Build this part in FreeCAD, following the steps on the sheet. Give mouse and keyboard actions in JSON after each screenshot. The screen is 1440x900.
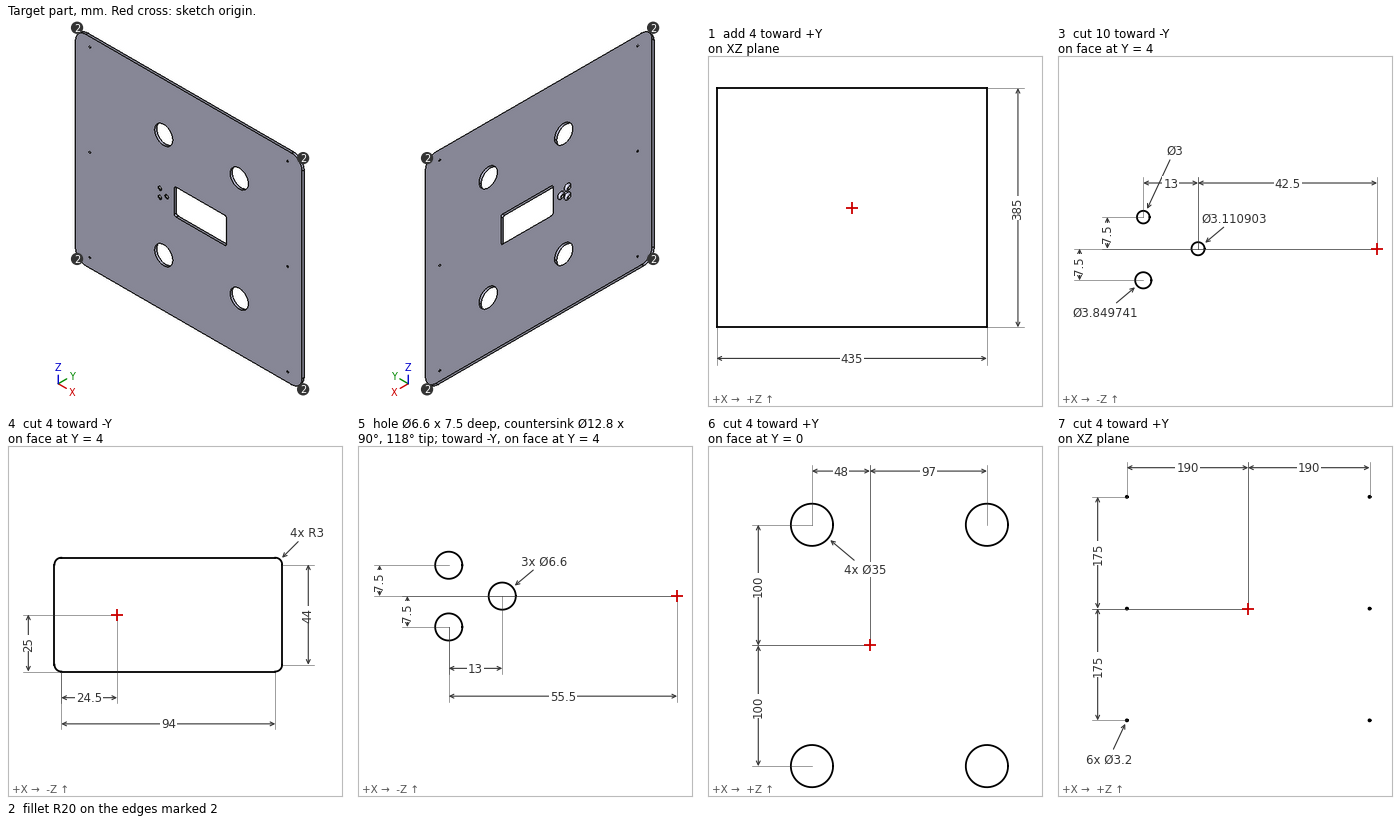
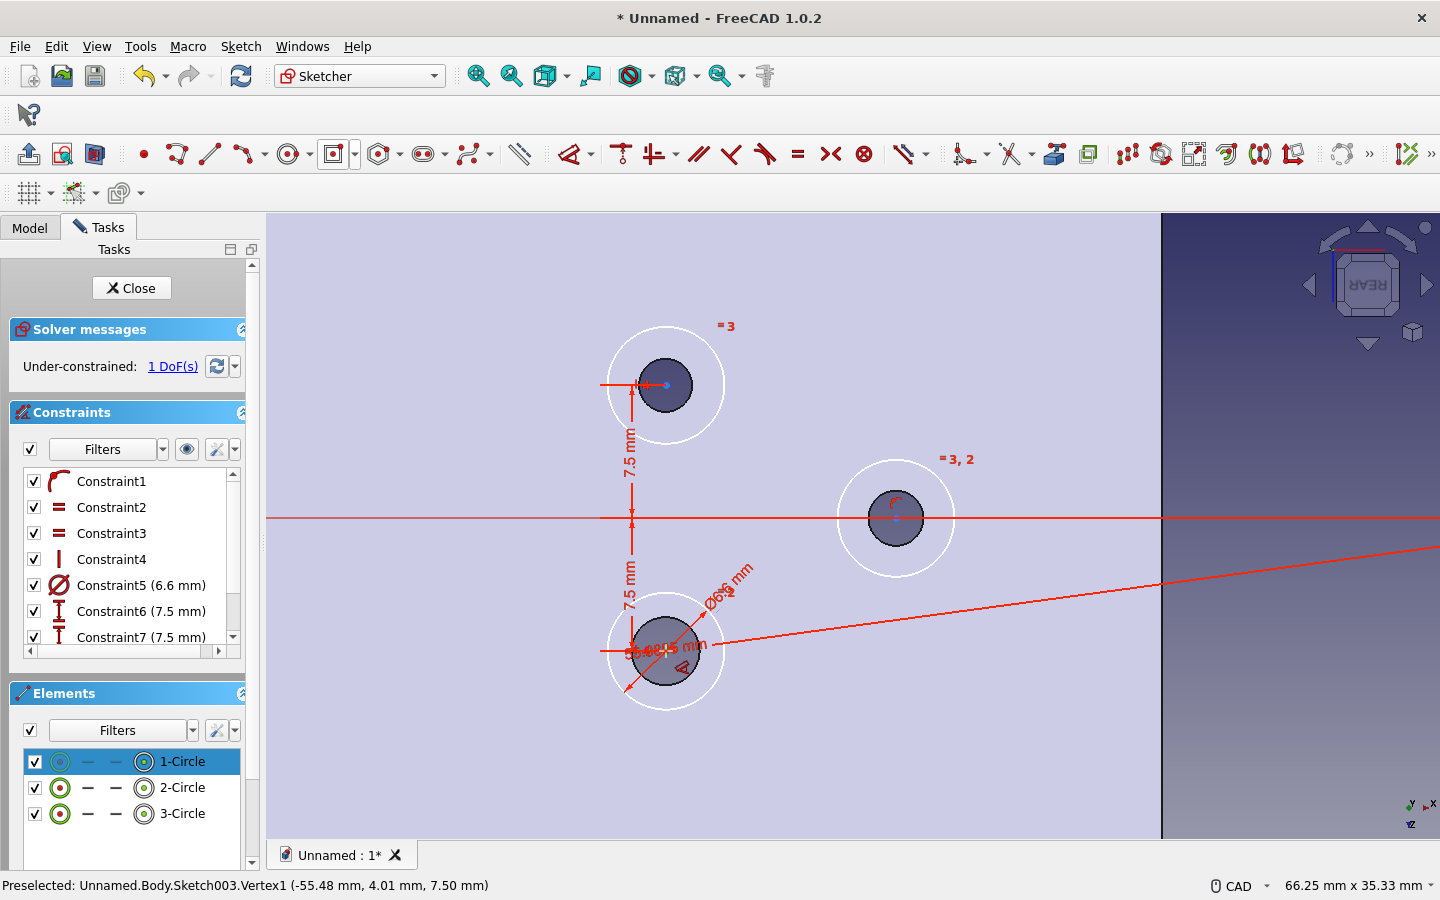
{"action": "left_click", "coordinate": [896, 518]}
{"action": "left_click", "coordinate": [781, 685]}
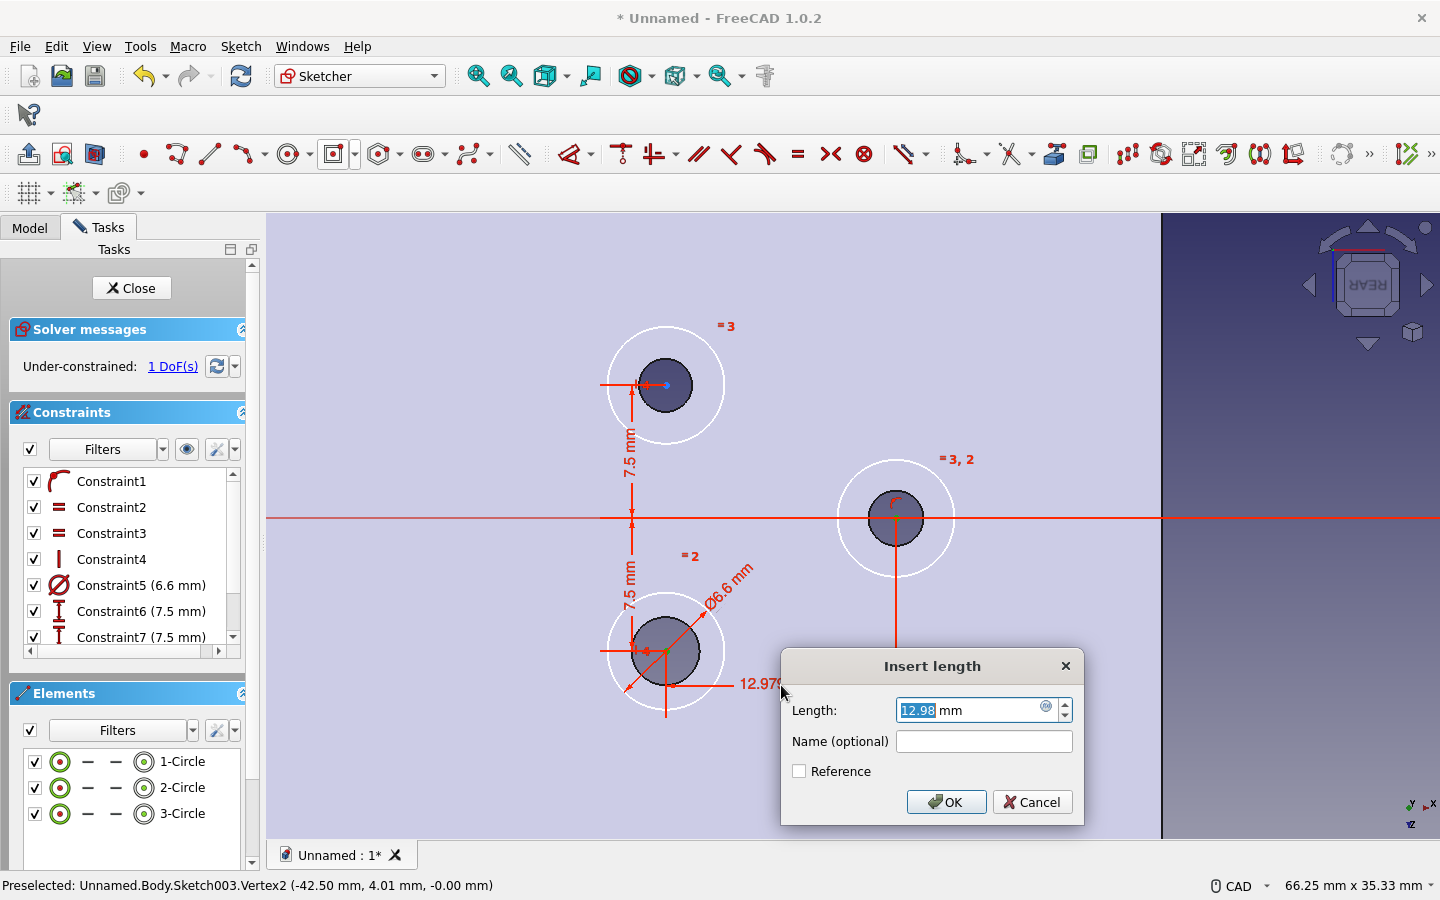
{"action": "type", "text": "13"}
{"action": "key", "text": "Return"}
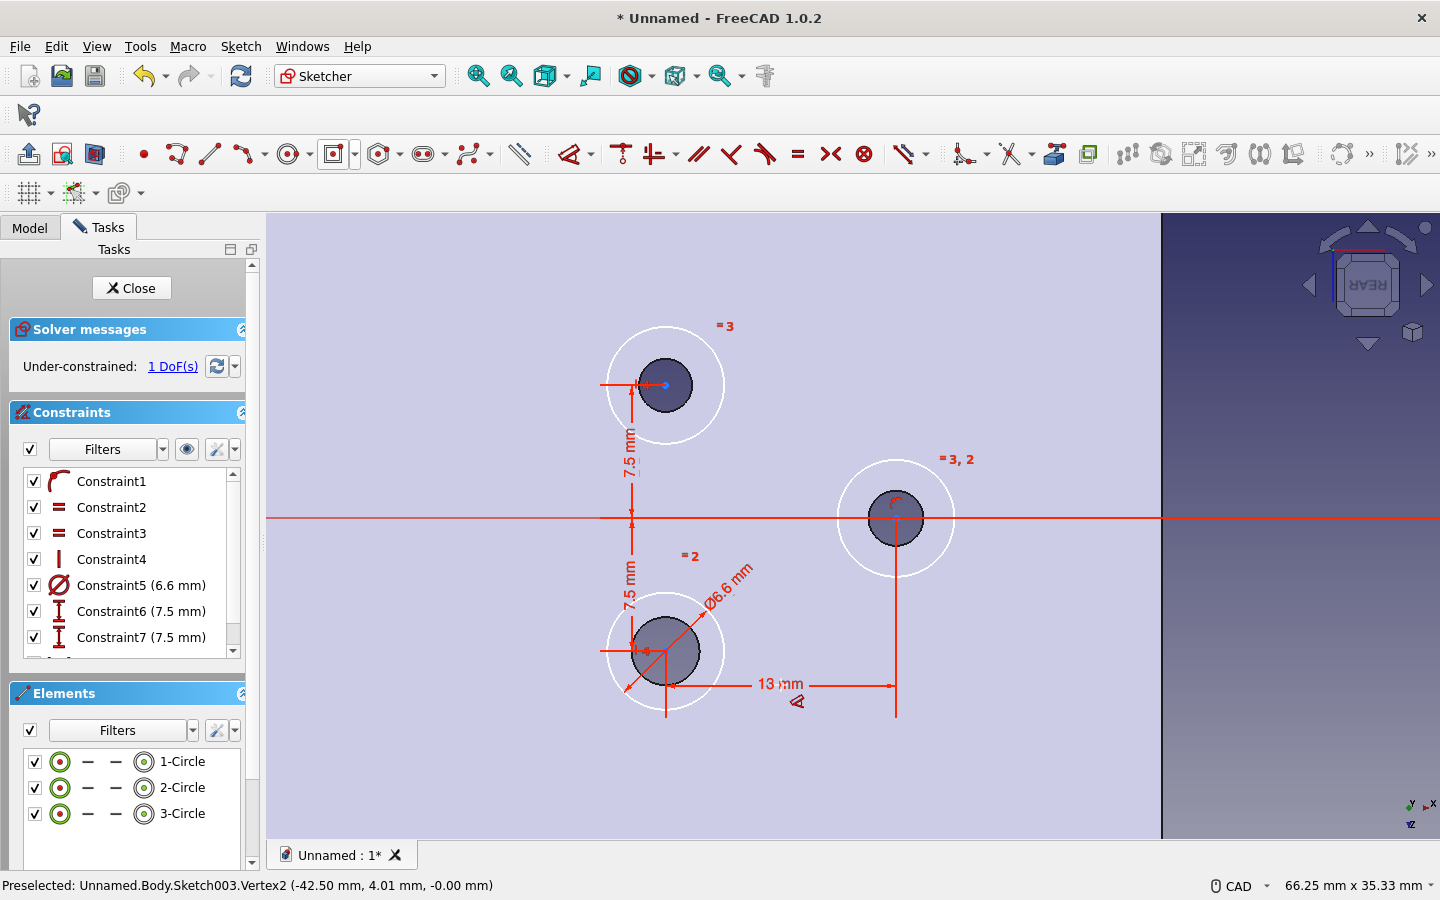
{"action": "left_click", "coordinate": [666, 651]}
{"action": "left_click", "coordinate": [970, 685]}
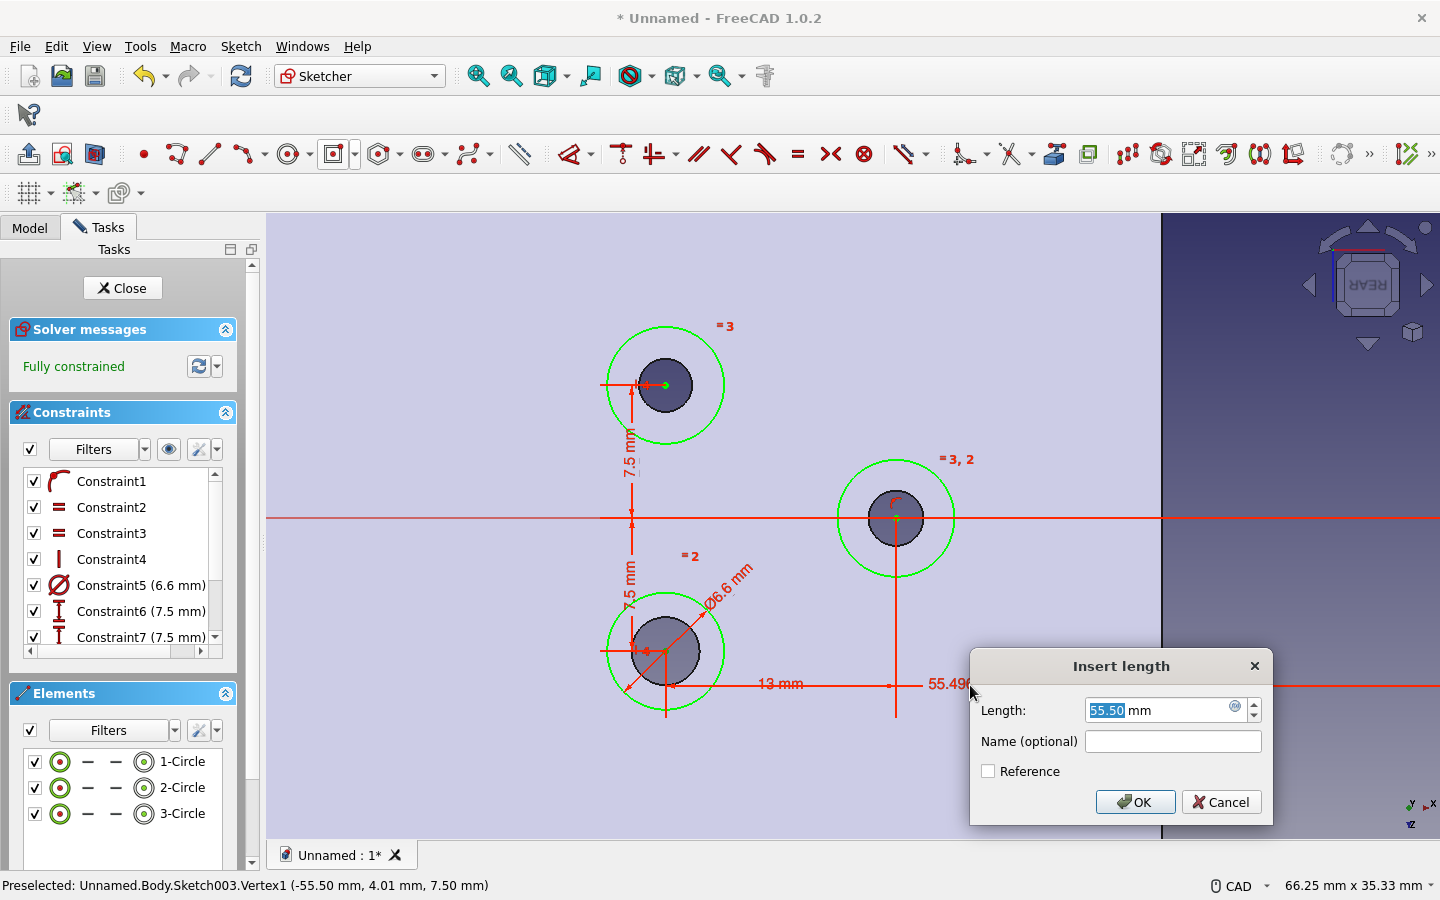
{"action": "type", "text": "55.5"}
{"action": "key", "text": "Return"}
{"action": "key", "text": "Escape"}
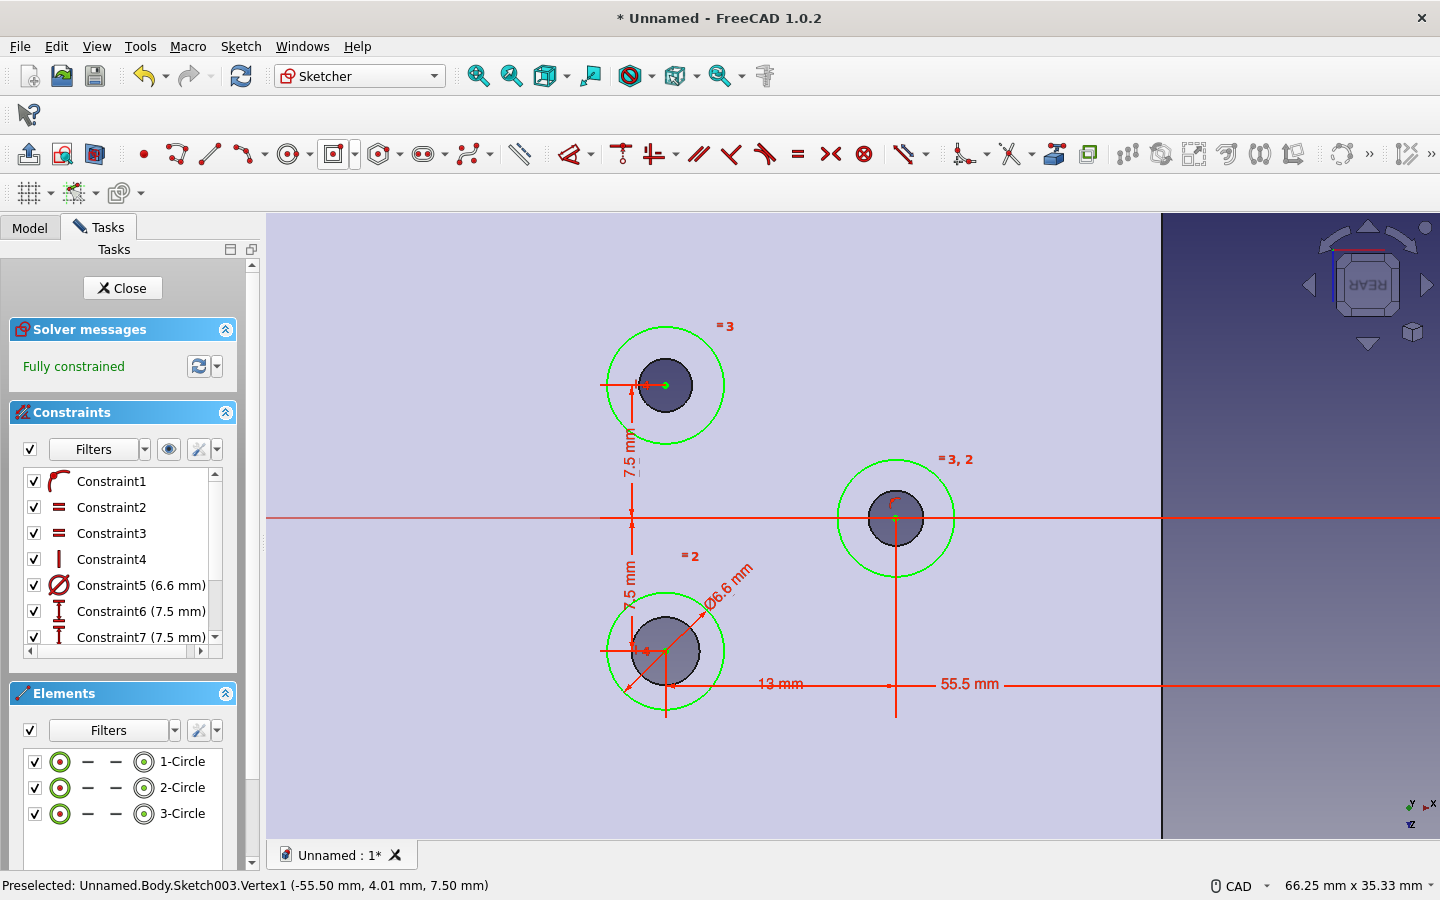
{"action": "left_click", "coordinate": [123, 288]}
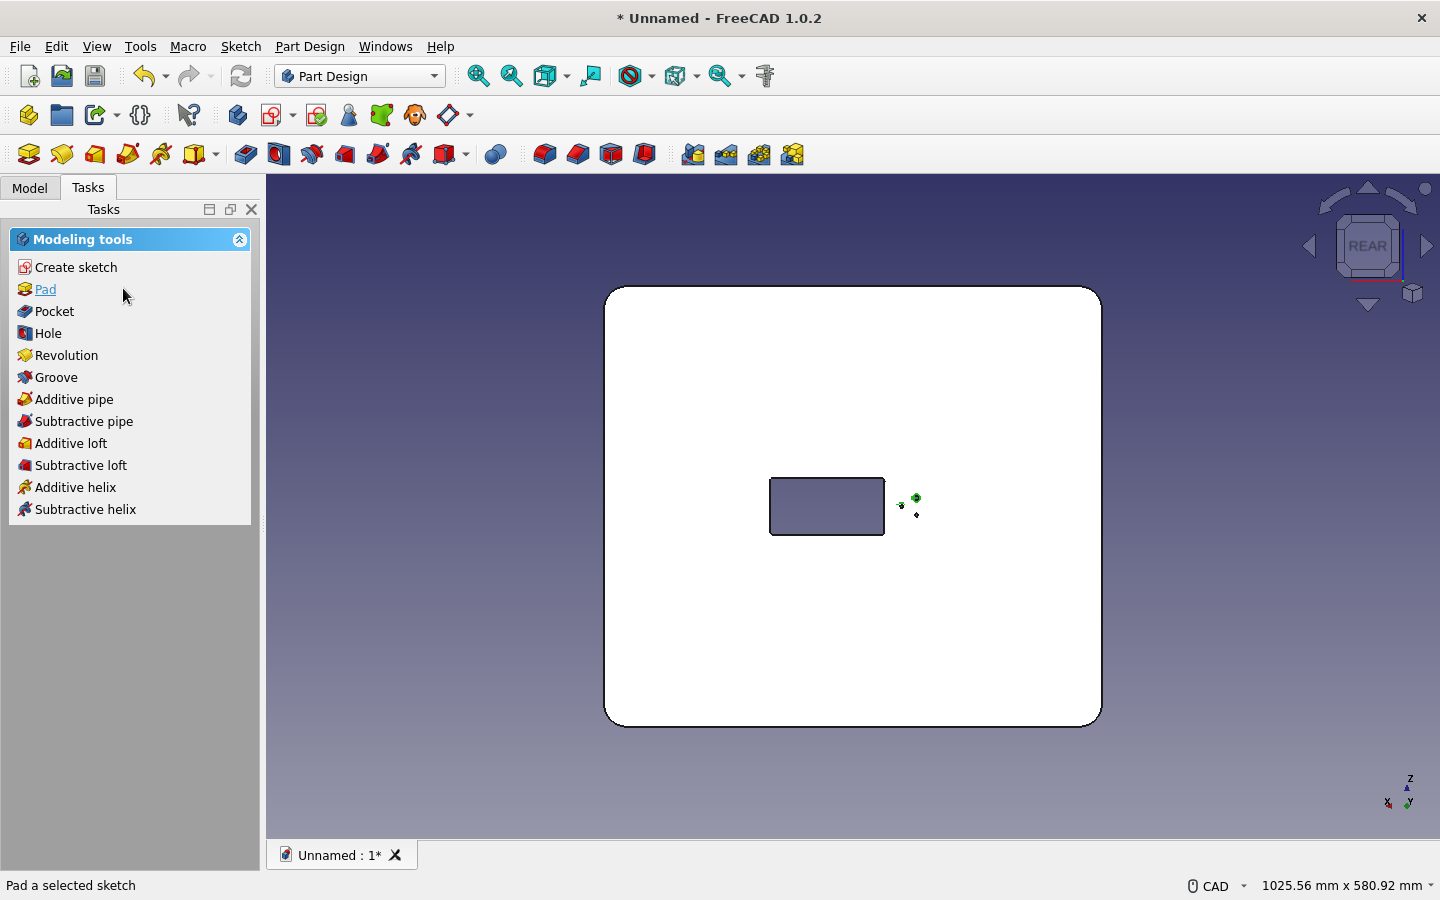
{"action": "left_click", "coordinate": [279, 154]}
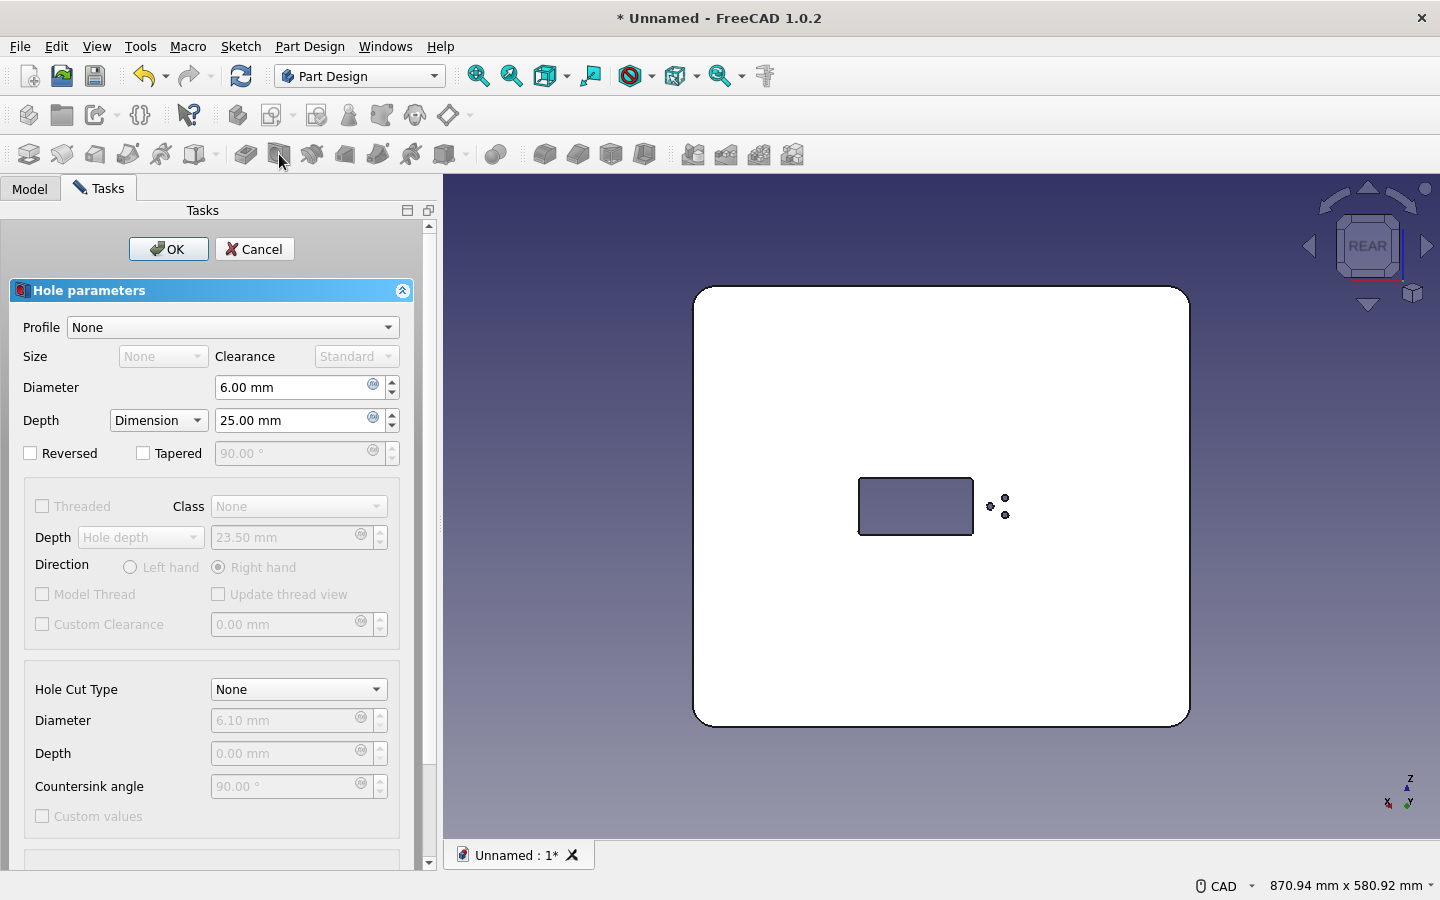
{"action": "triple_click", "coordinate": [300, 388]}